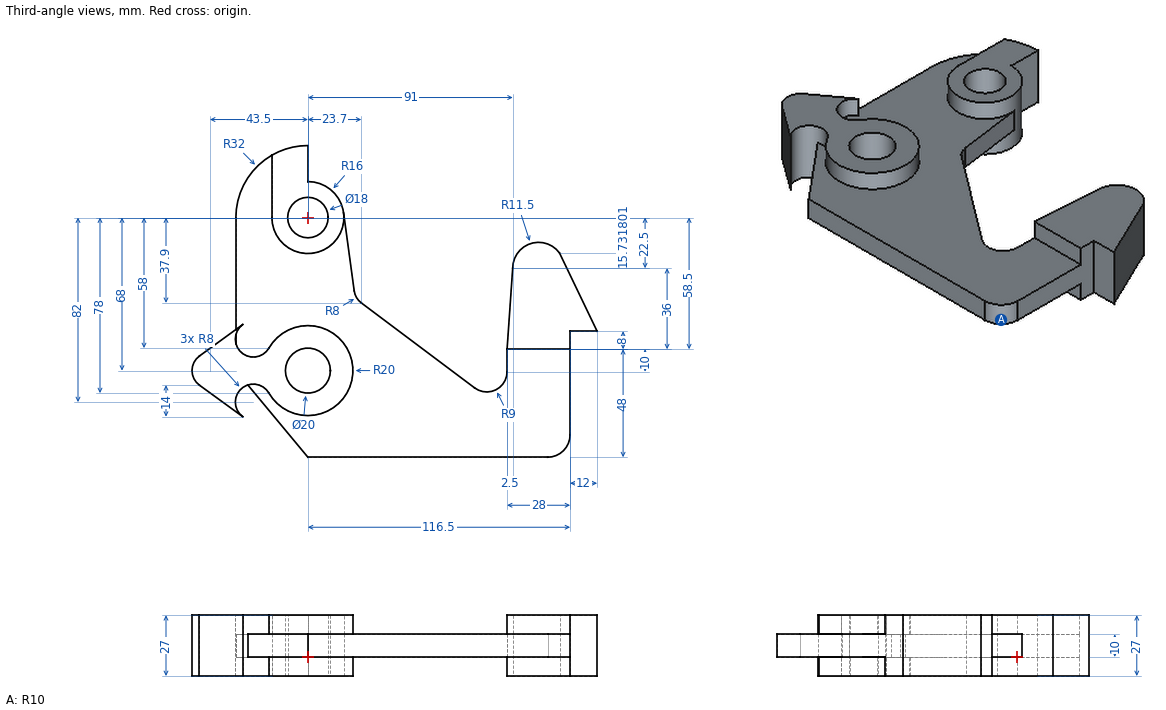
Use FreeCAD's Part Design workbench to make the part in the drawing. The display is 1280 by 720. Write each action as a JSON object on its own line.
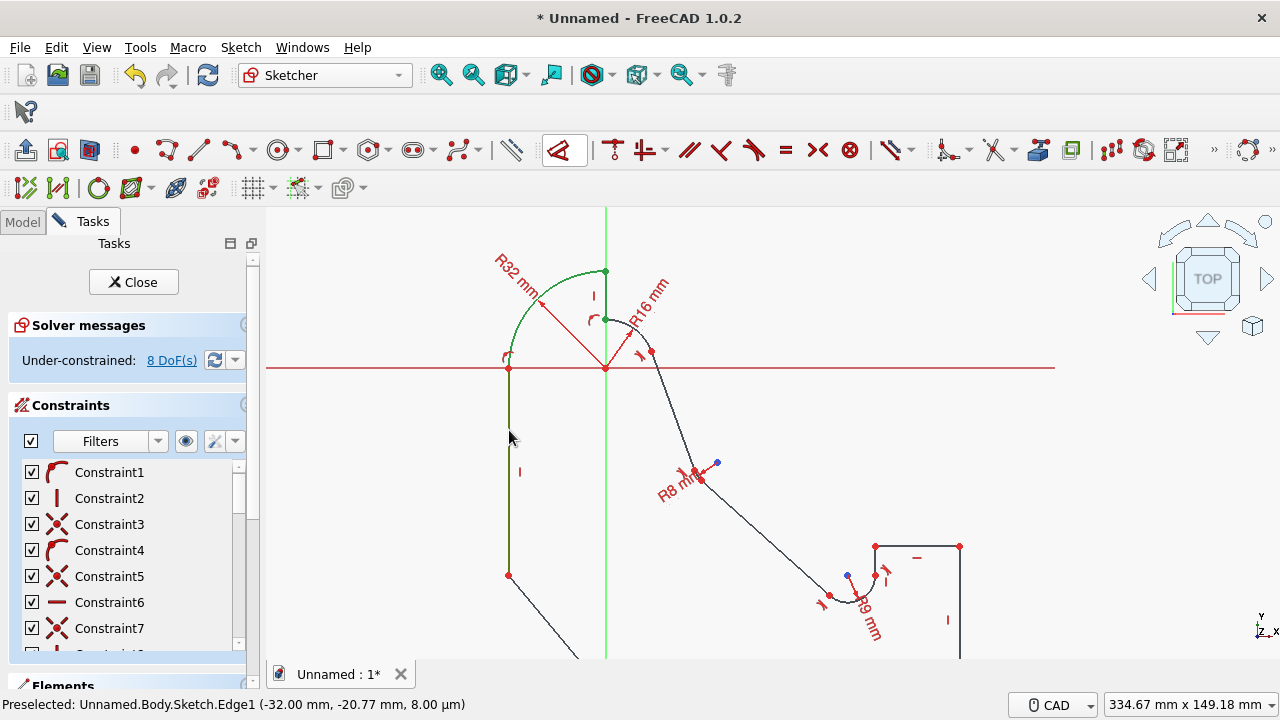
{"action": "key", "text": "i"}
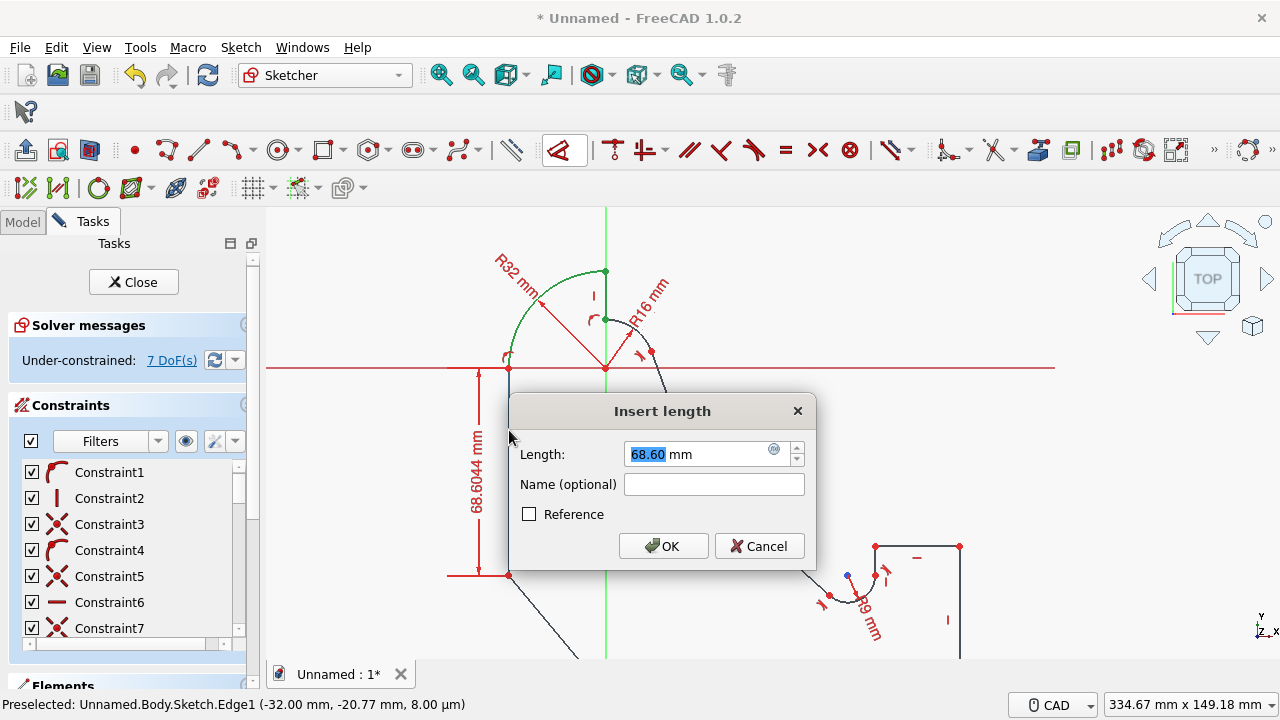
{"action": "type", "text": "68"}
{"action": "key", "text": "Return"}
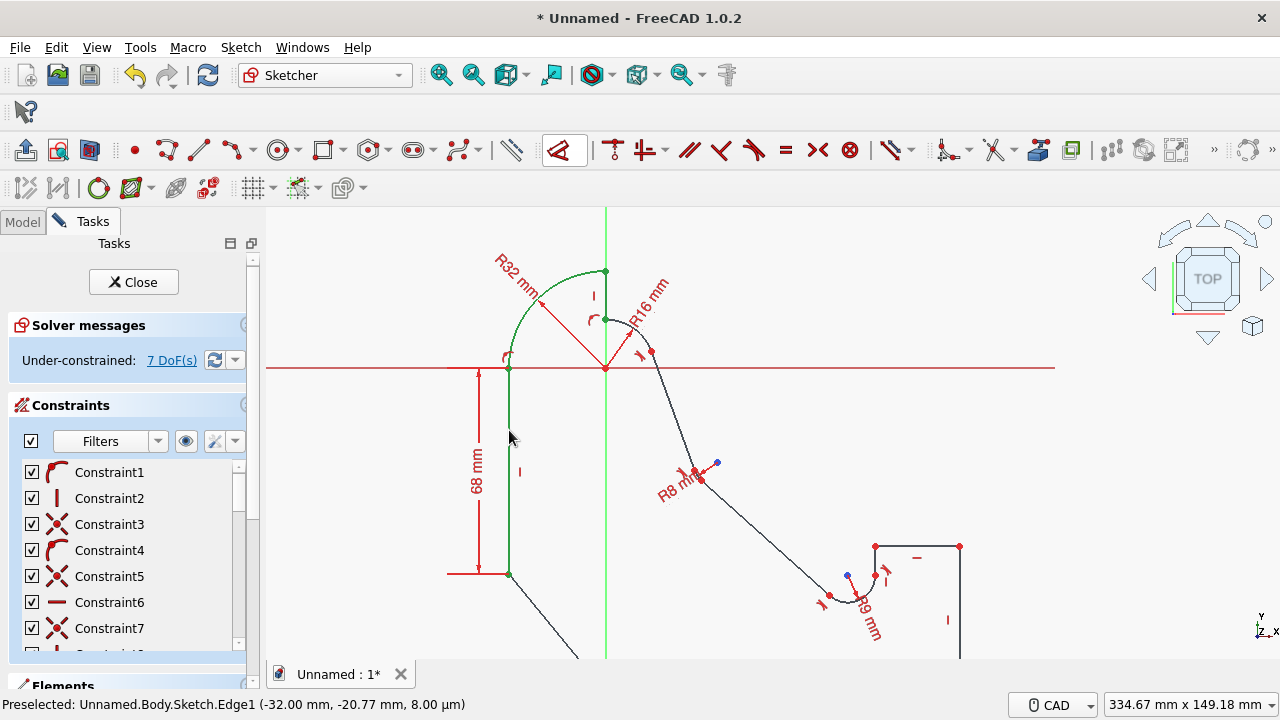
{"action": "left_click", "coordinate": [960, 590]}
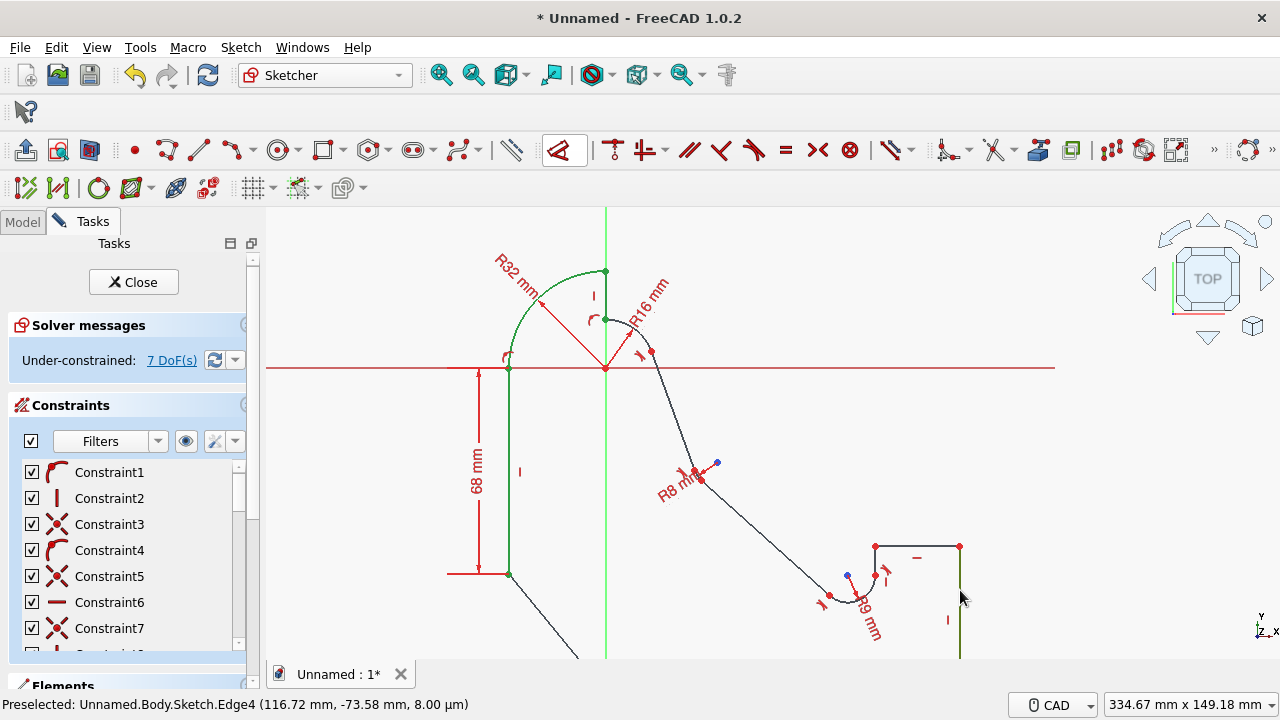
{"action": "left_click", "coordinate": [582, 150]}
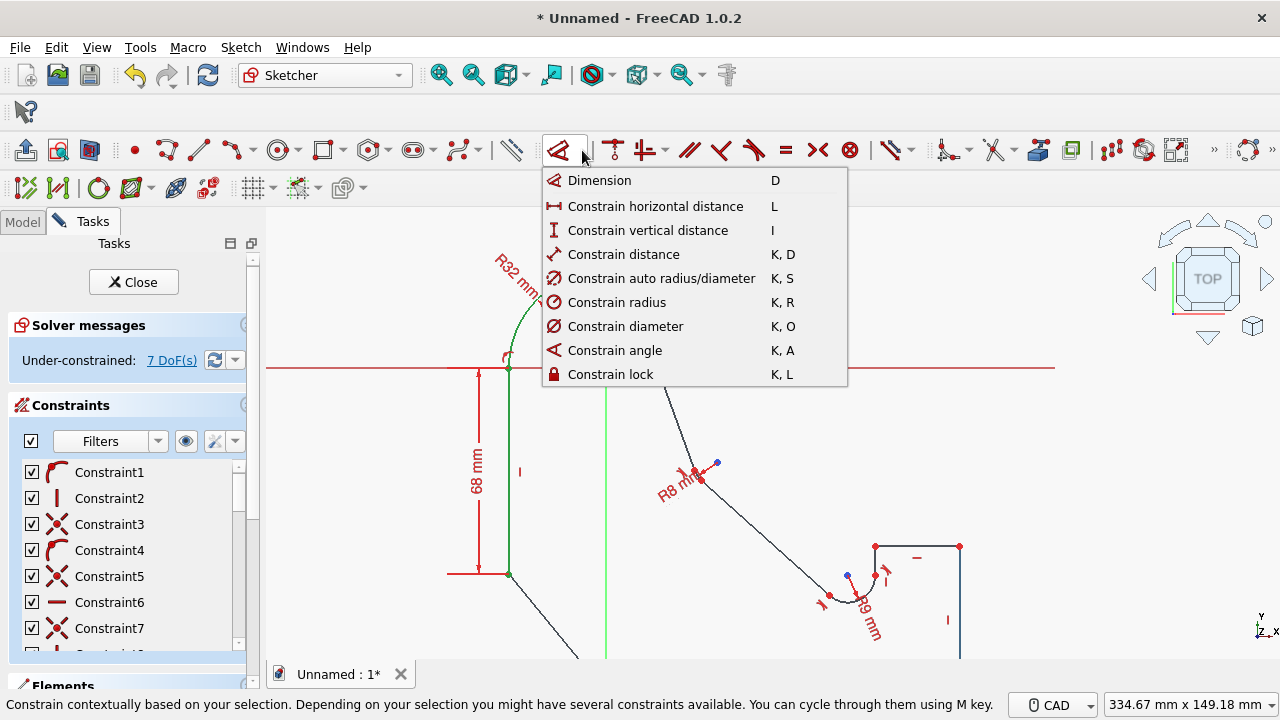
{"action": "left_click", "coordinate": [695, 230]}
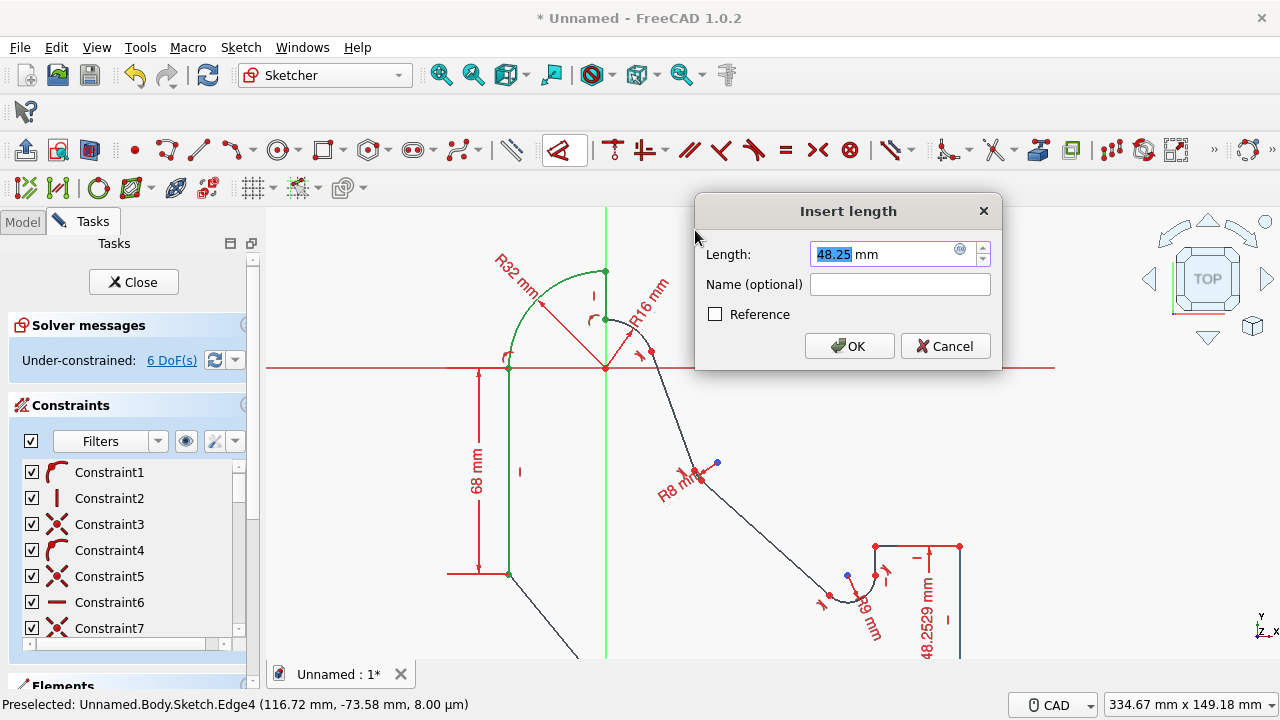
{"action": "type", "text": "48"}
{"action": "key", "text": "Return"}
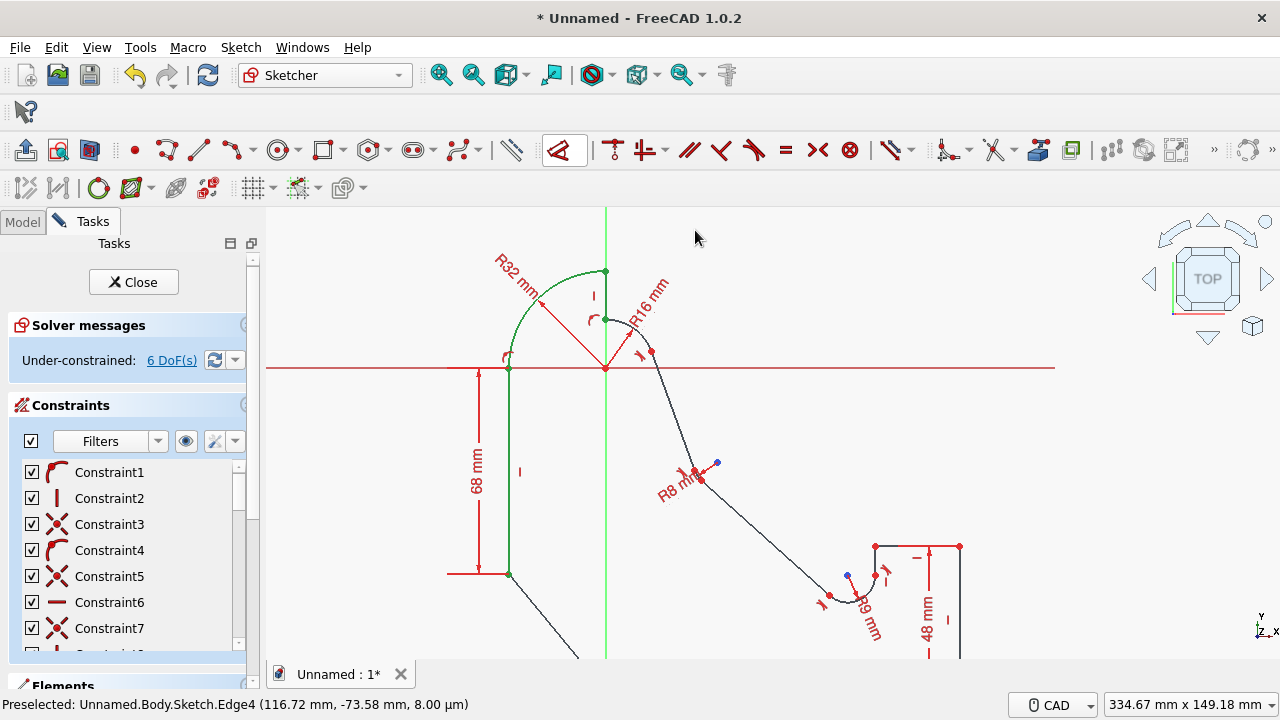
{"action": "left_click", "coordinate": [934, 546]}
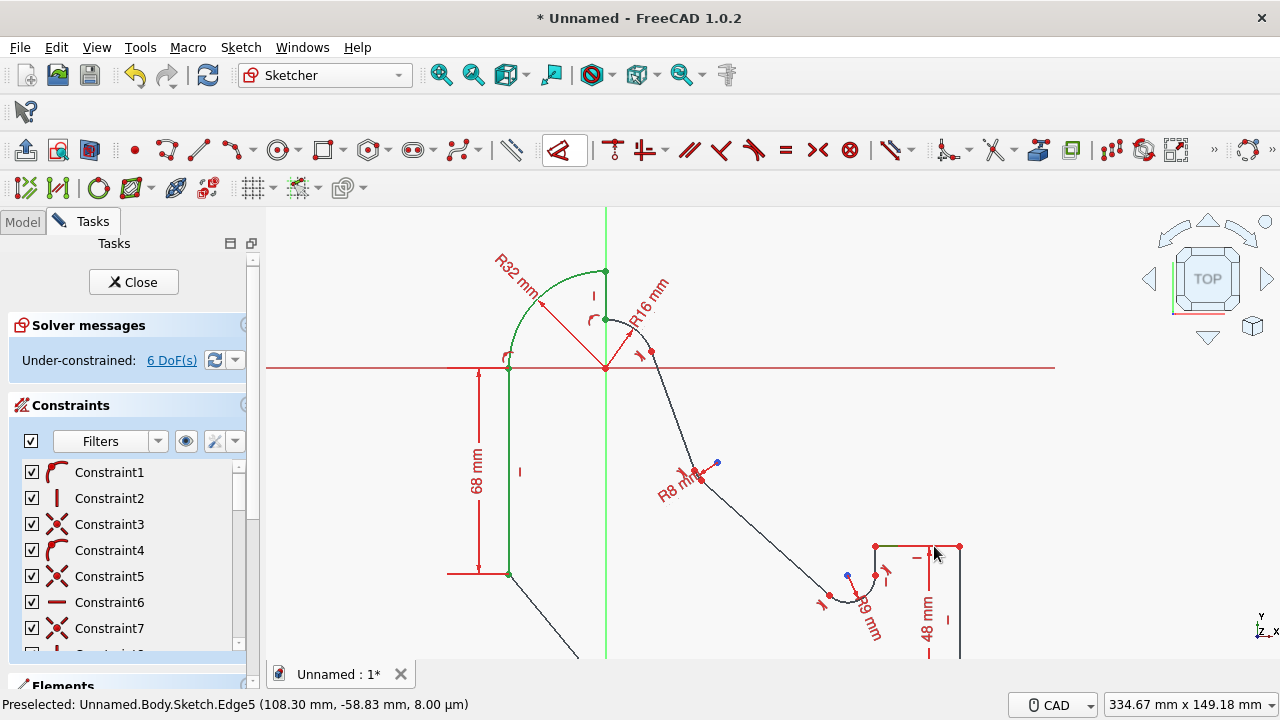
{"action": "key", "text": "l"}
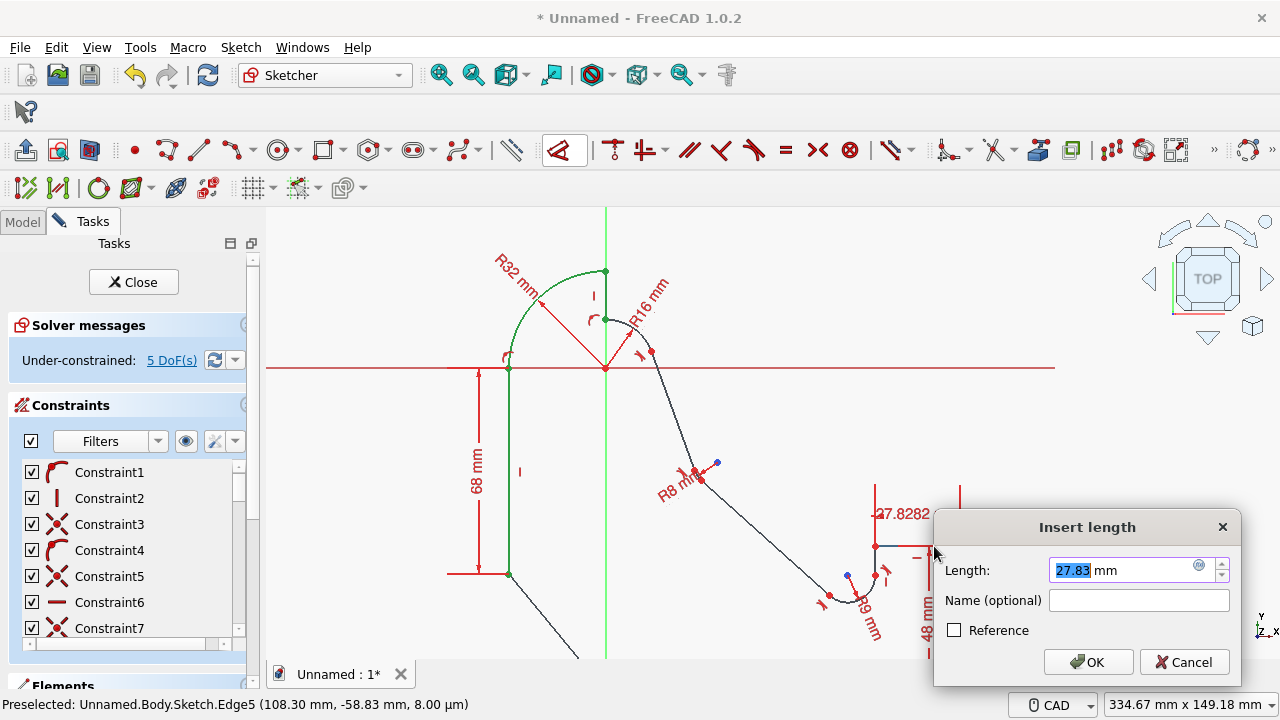
{"action": "type", "text": "28"}
{"action": "key", "text": "Return"}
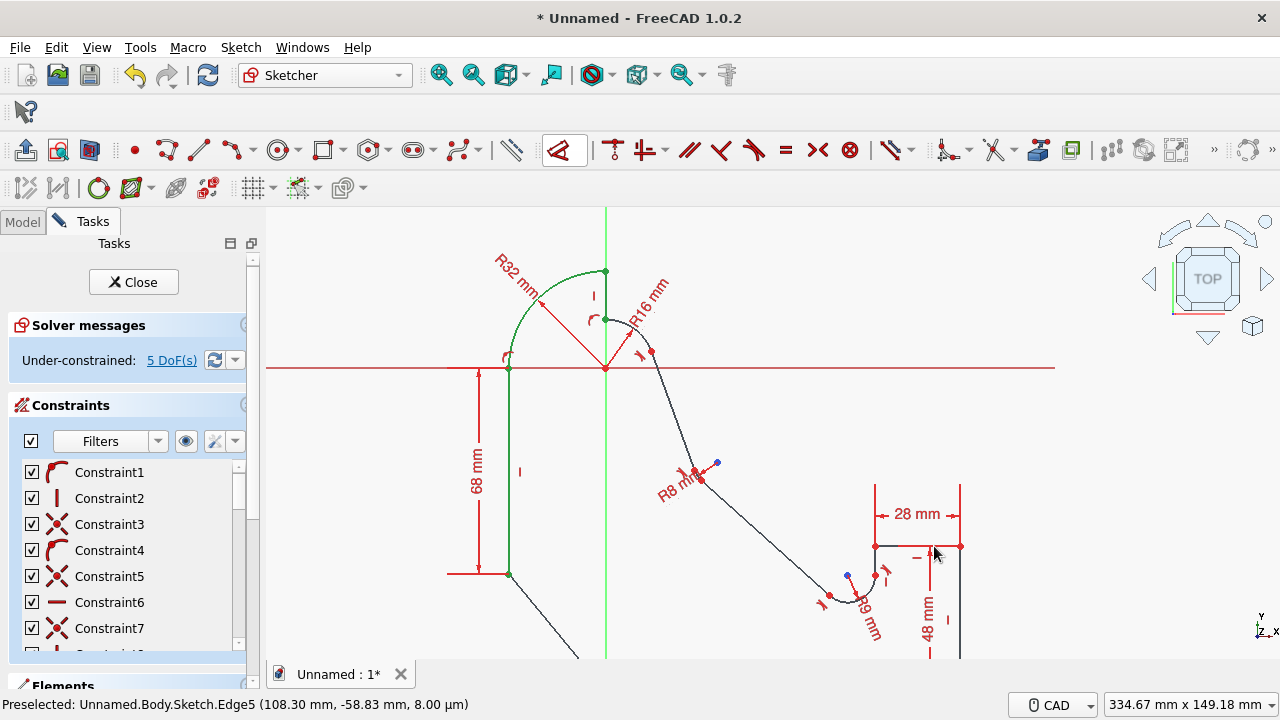
{"action": "scroll", "coordinate": [875, 558], "scroll_direction": "up", "scroll_amount": 2}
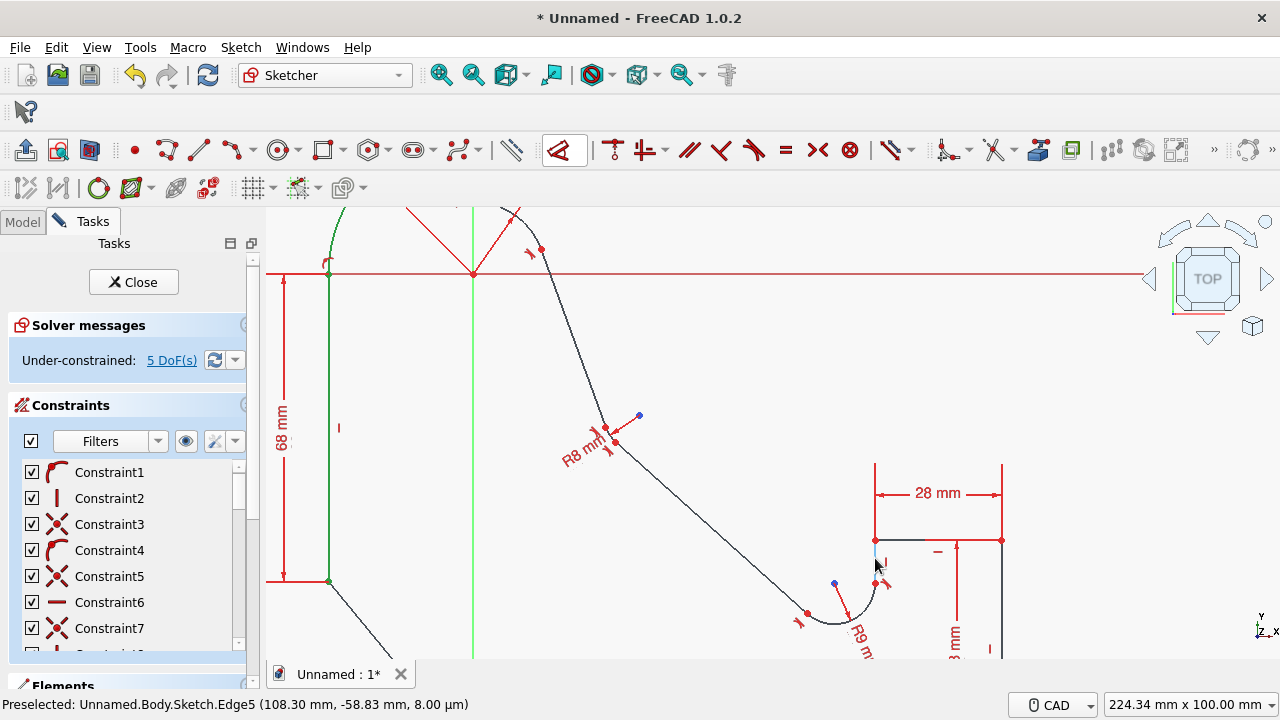
{"action": "left_click", "coordinate": [875, 557]}